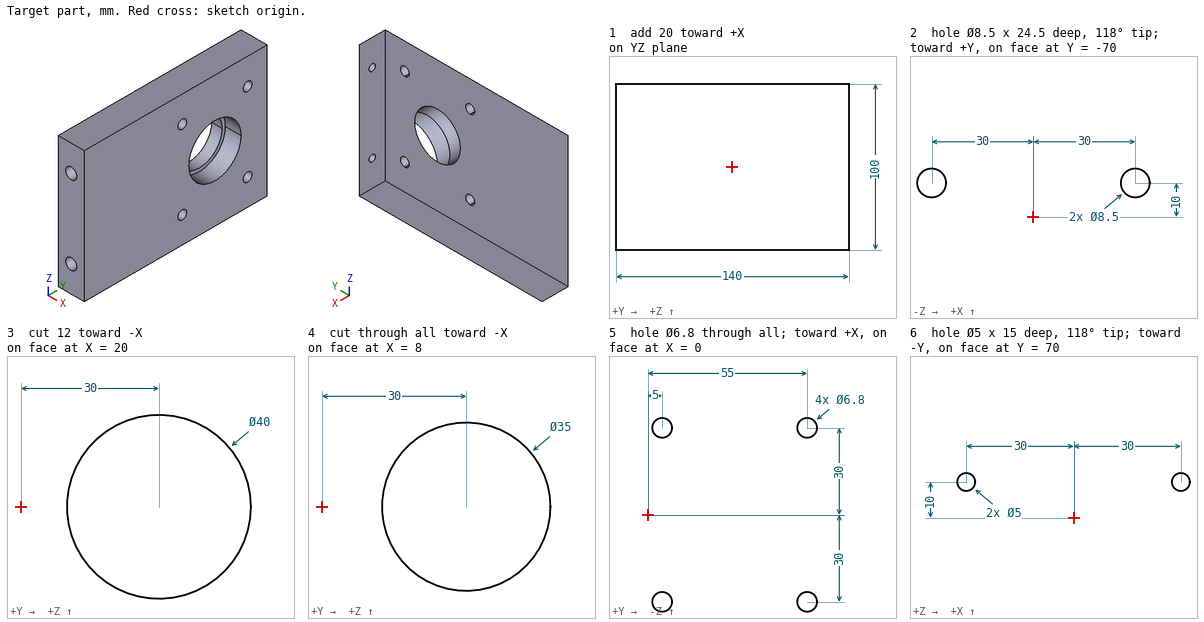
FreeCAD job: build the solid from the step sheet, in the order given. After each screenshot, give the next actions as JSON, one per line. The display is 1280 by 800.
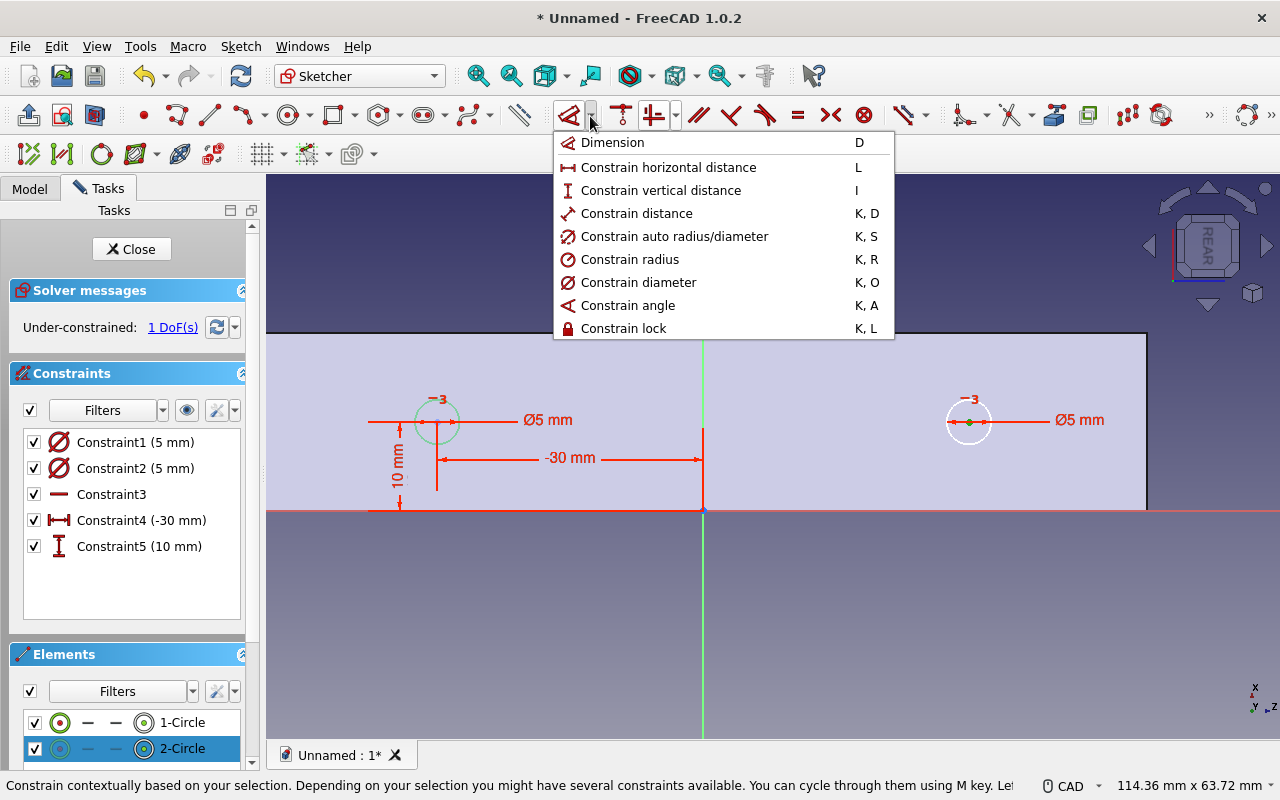
{"action": "left_click", "coordinate": [724, 168]}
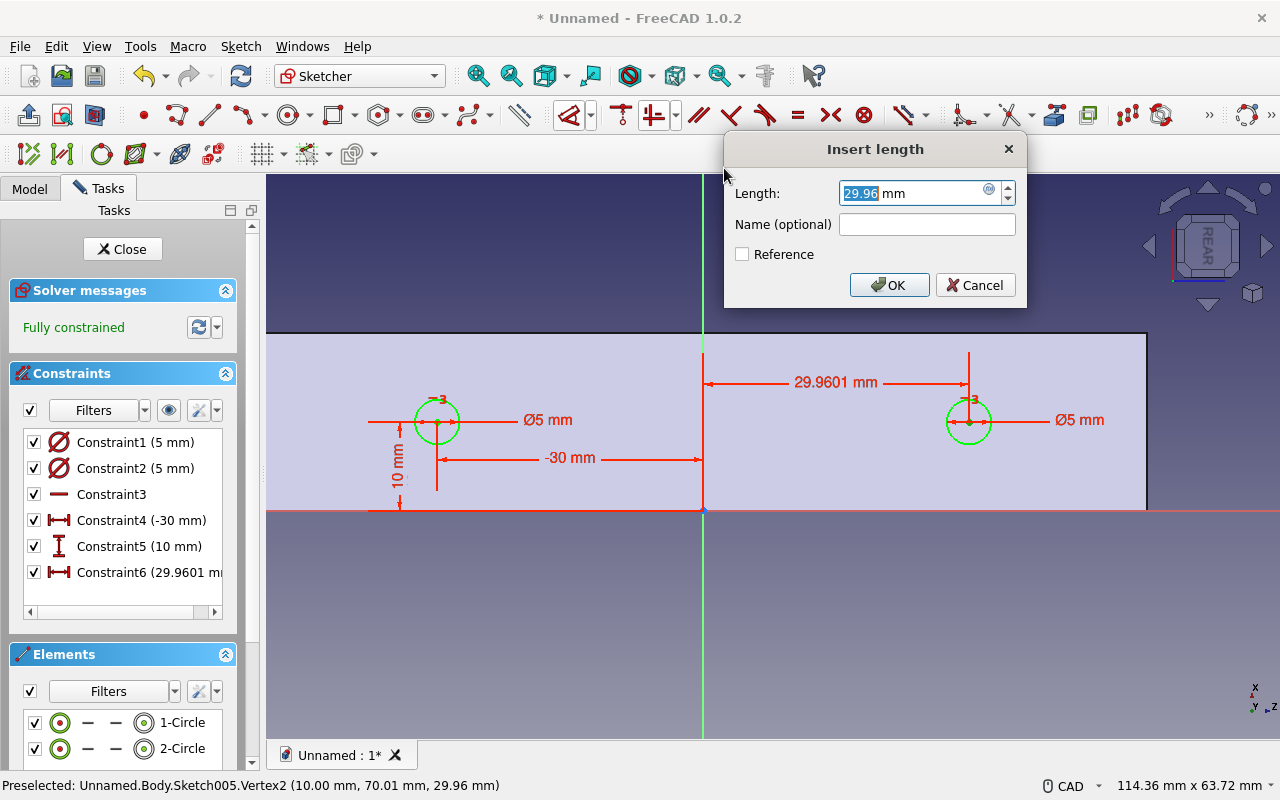
{"action": "type", "text": "30"}
{"action": "key", "text": "Return"}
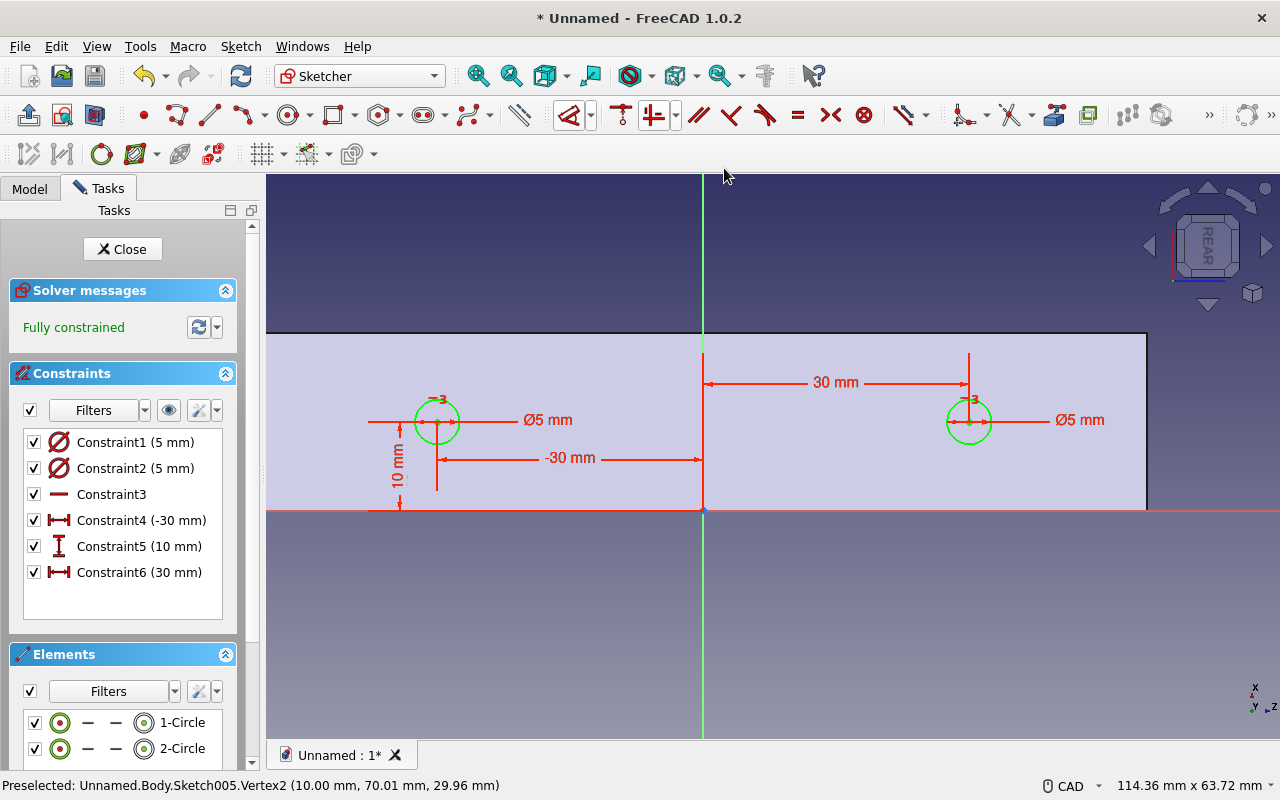
{"action": "left_click", "coordinate": [123, 249]}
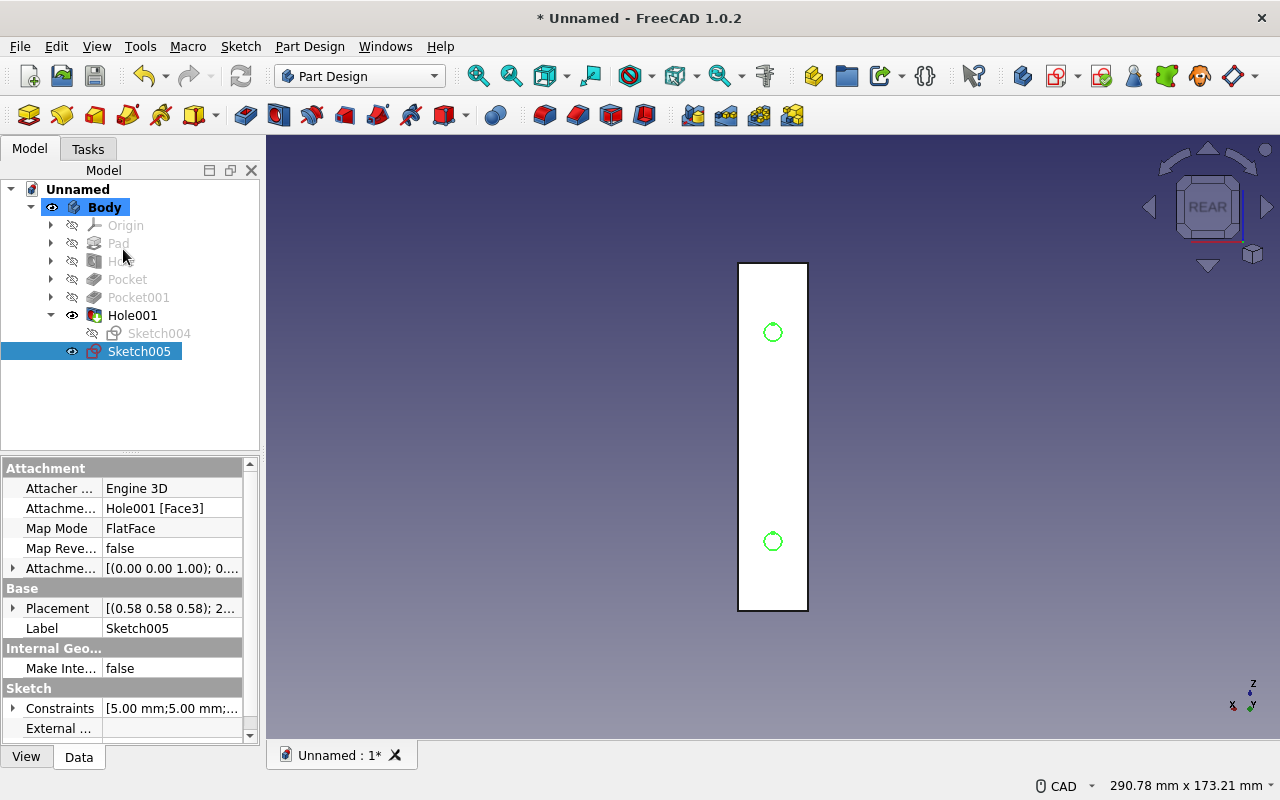
{"action": "left_click", "coordinate": [279, 116]}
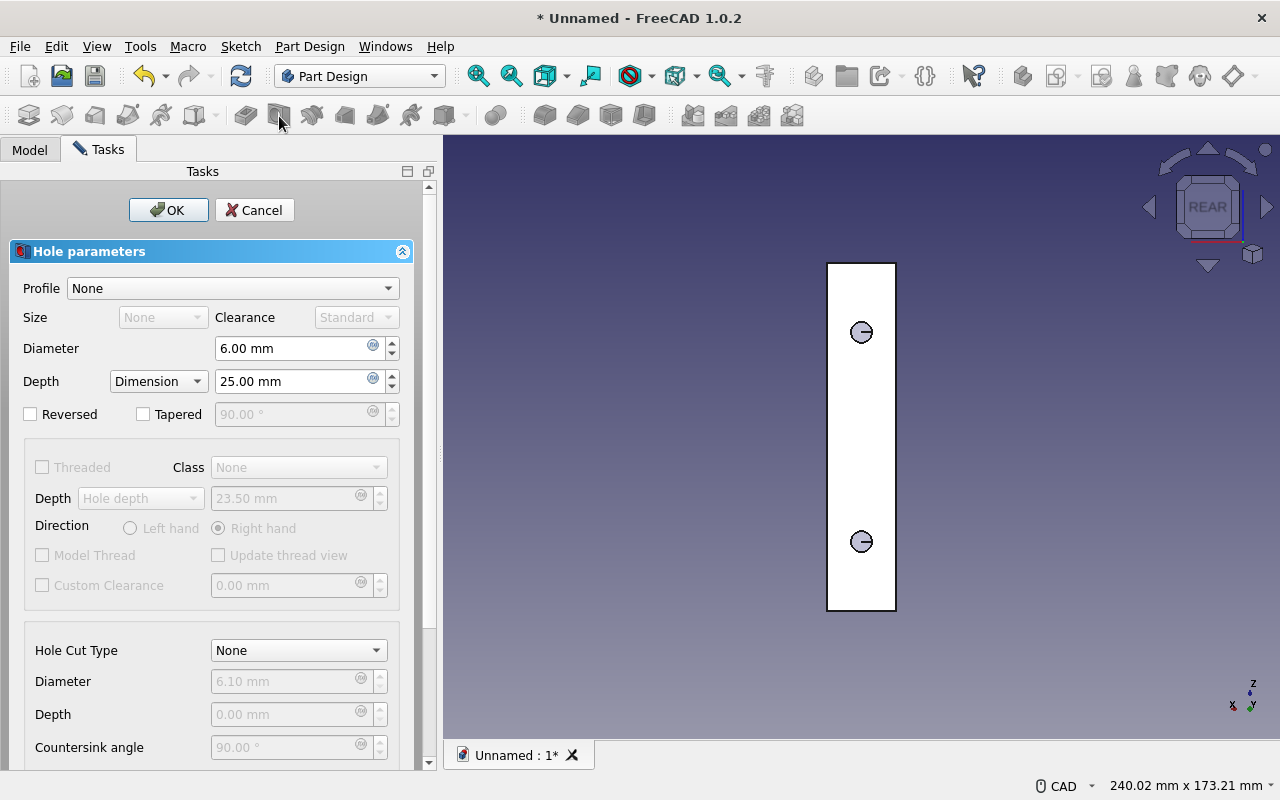
{"action": "triple_click", "coordinate": [300, 348]}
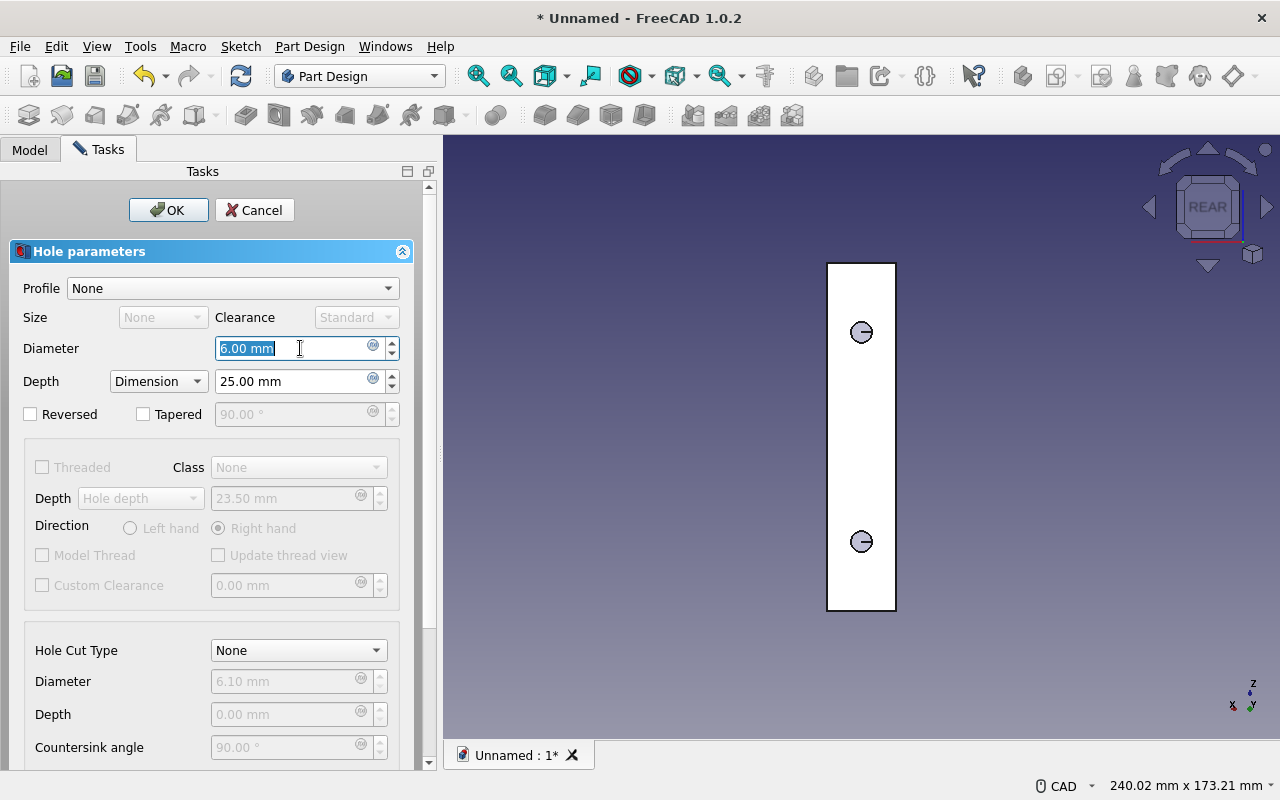
{"action": "type", "text": "5"}
{"action": "key", "text": "Tab"}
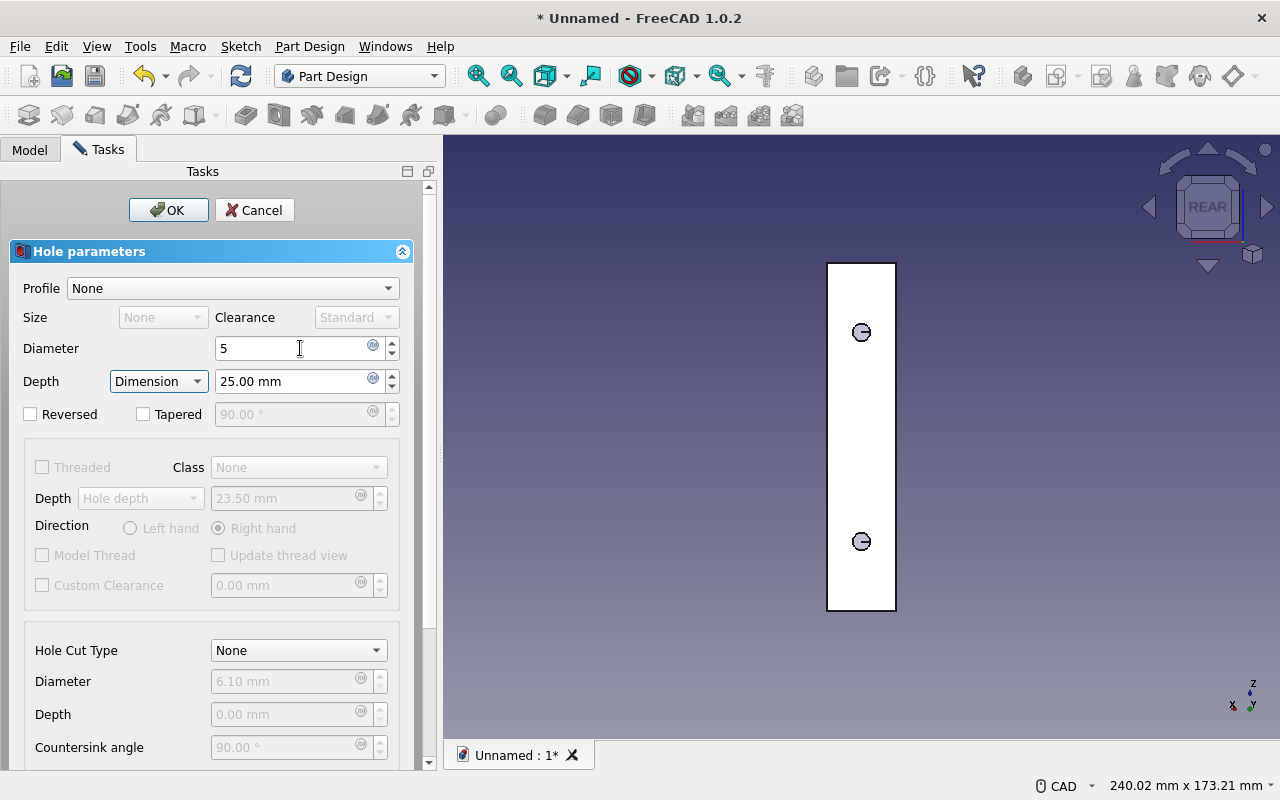
{"action": "triple_click", "coordinate": [300, 382]}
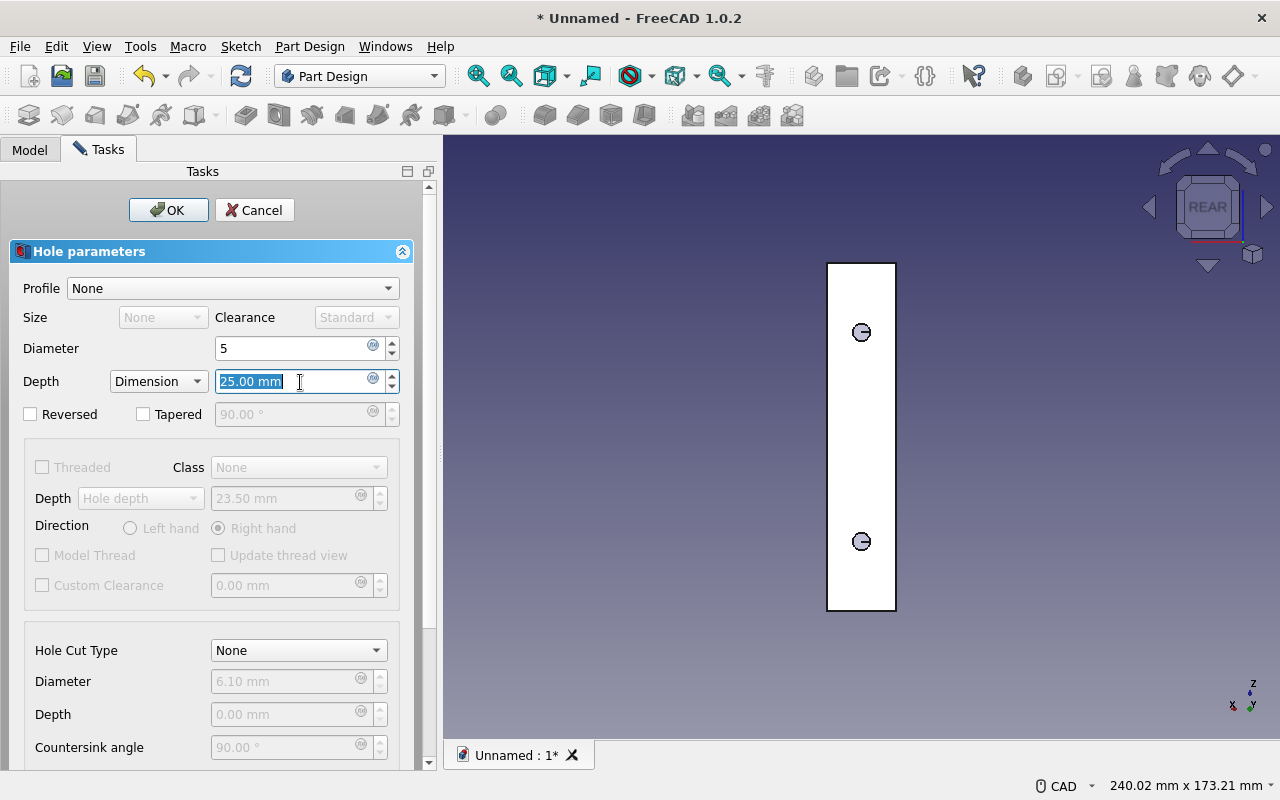
{"action": "type", "text": "15"}
{"action": "key", "text": "Tab"}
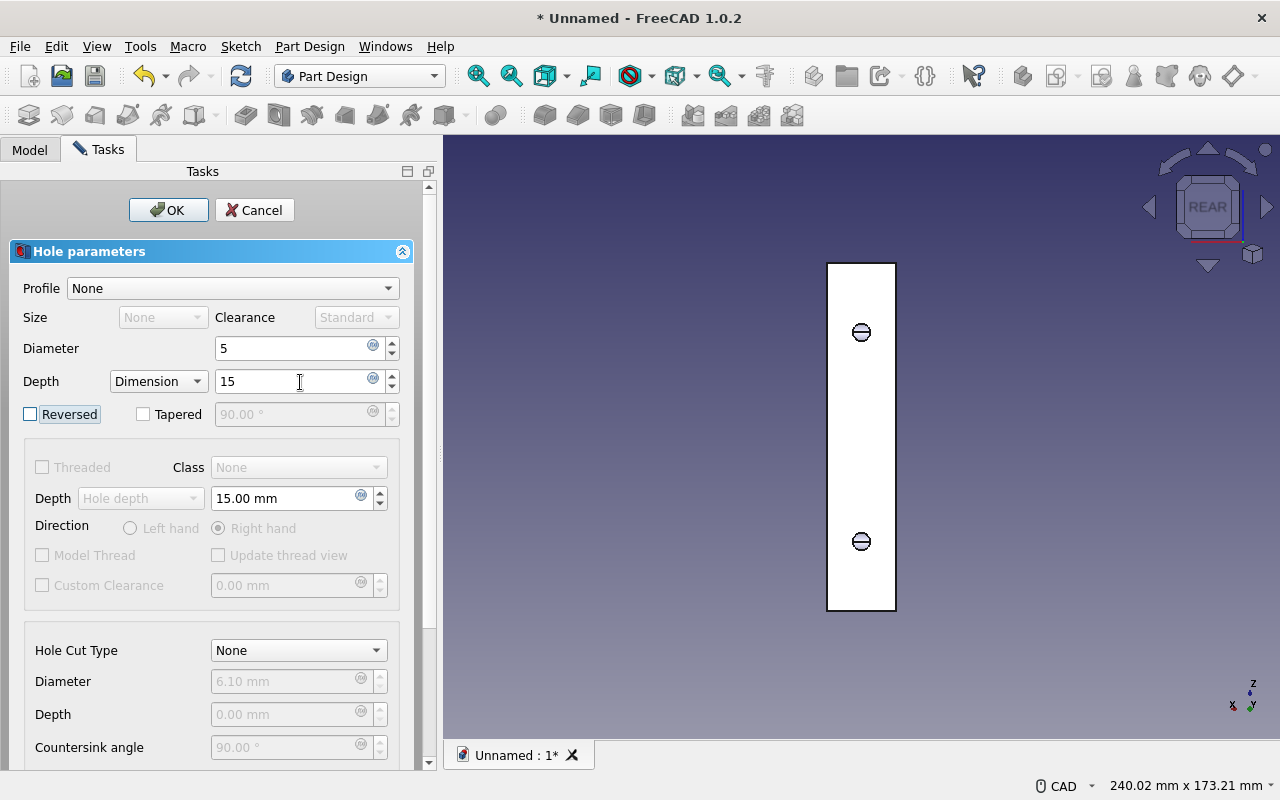
{"action": "left_click", "coordinate": [169, 210]}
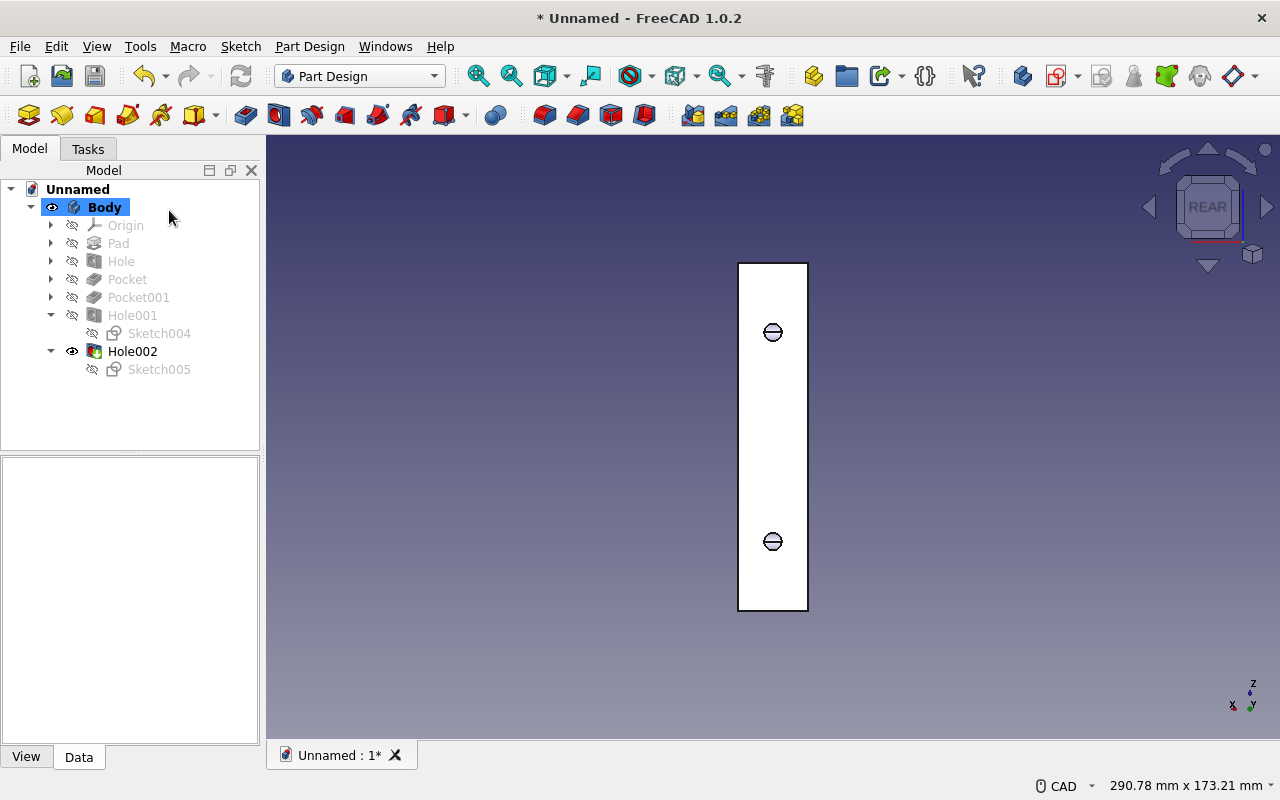
{"action": "key", "text": "0"}